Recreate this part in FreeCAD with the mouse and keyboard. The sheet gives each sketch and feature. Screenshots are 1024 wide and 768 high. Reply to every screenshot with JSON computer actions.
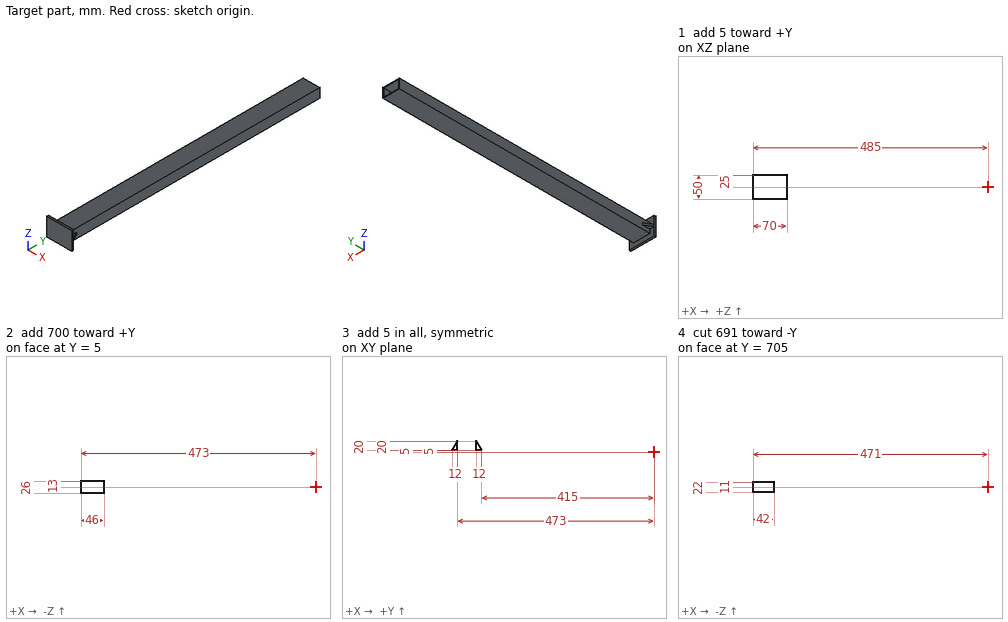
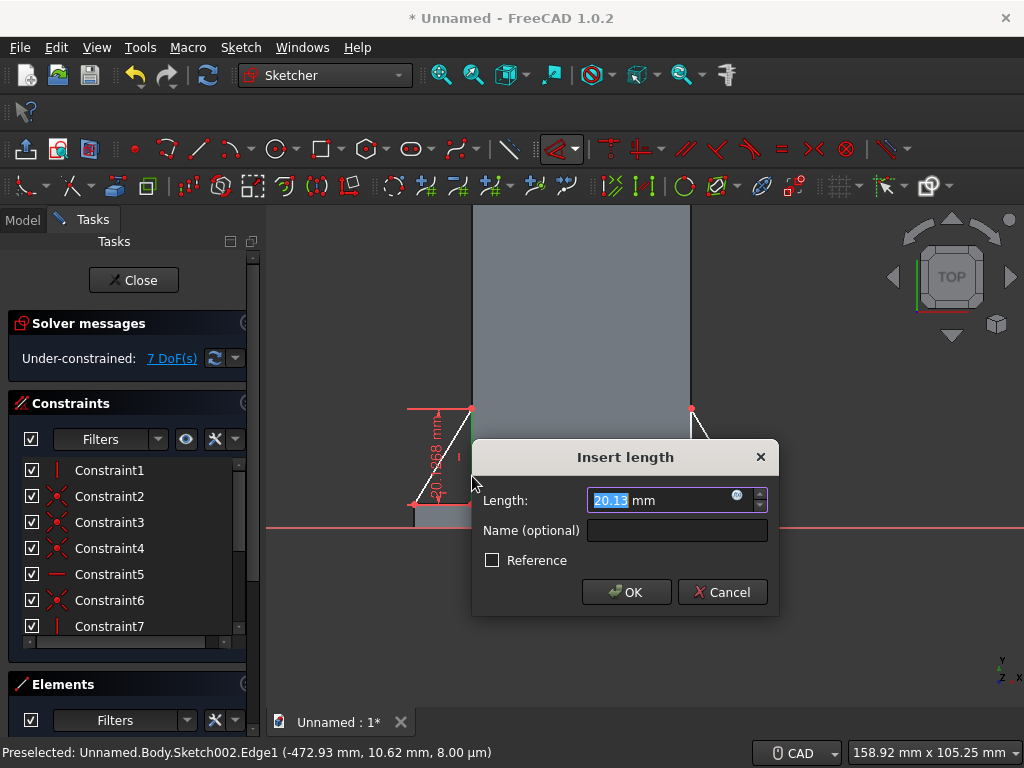
{"action": "type", "text": "20"}
{"action": "key", "text": "Return"}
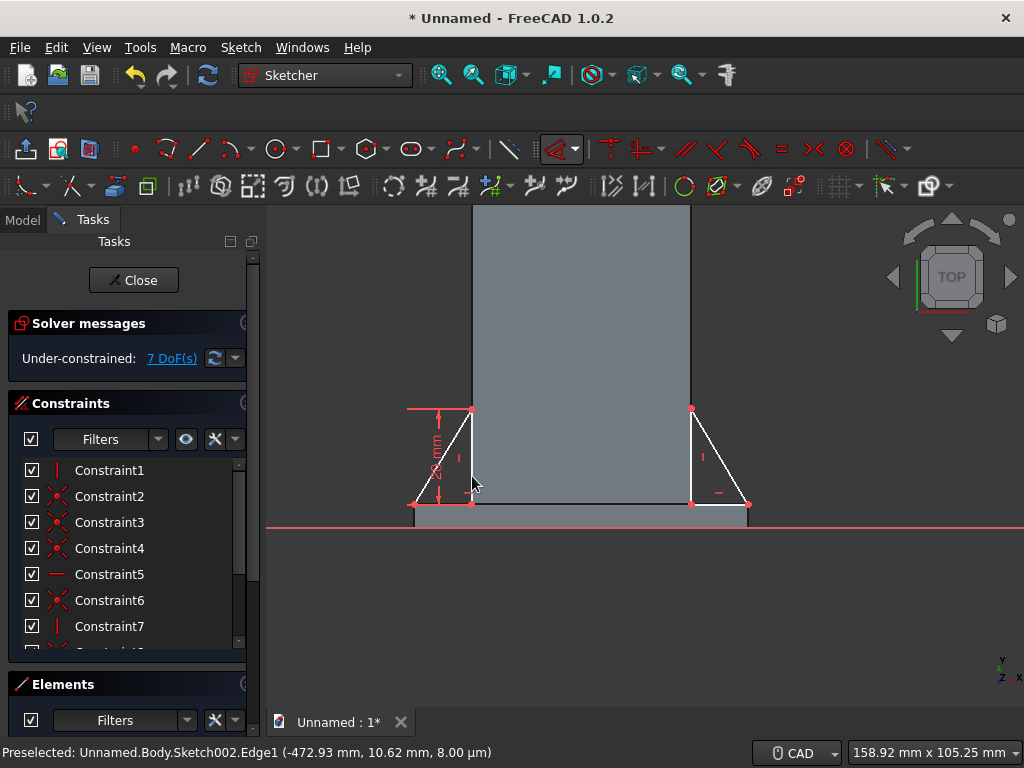
{"action": "left_click", "coordinate": [431, 505]}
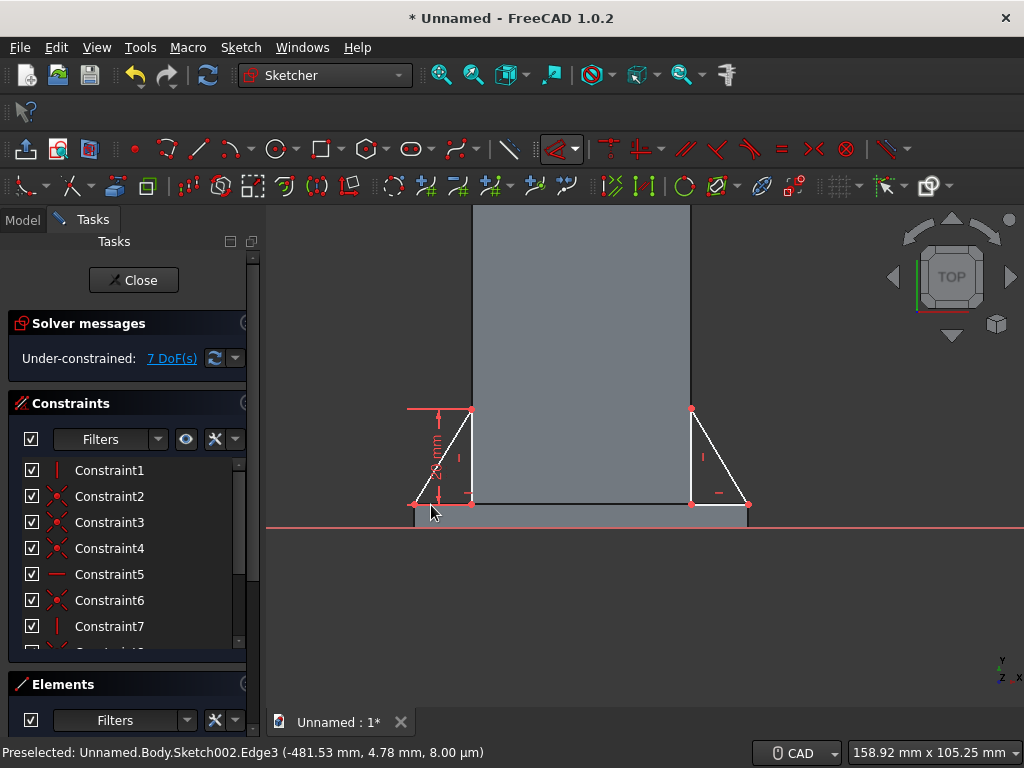
{"action": "key", "text": "l"}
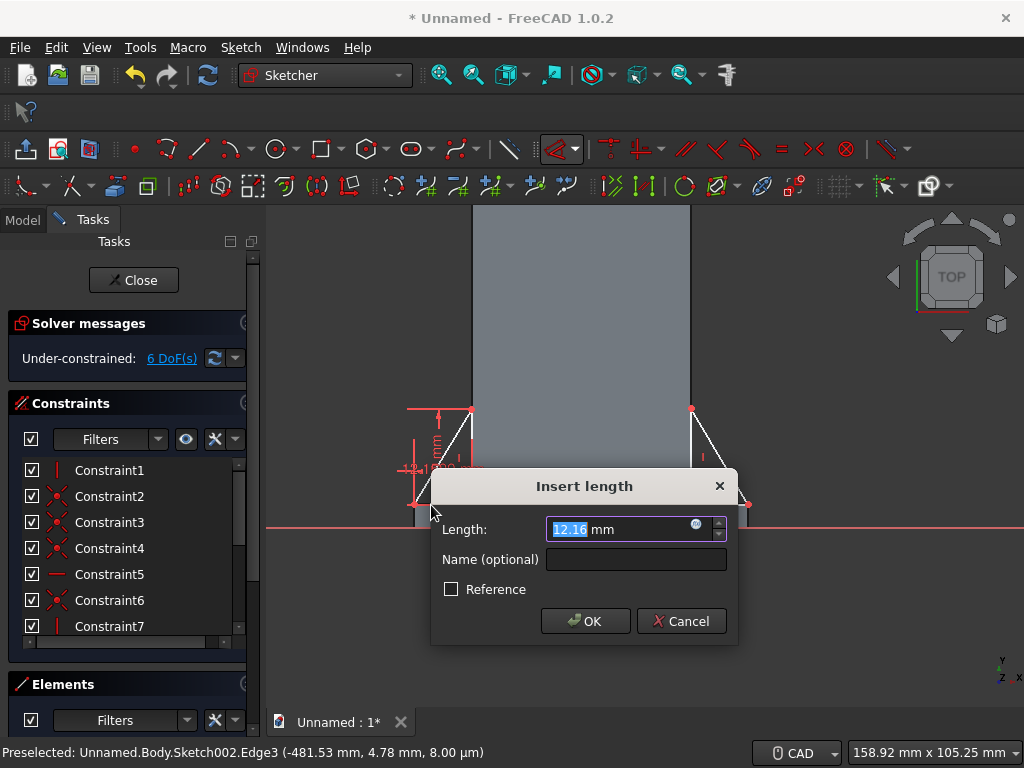
{"action": "type", "text": "12"}
{"action": "key", "text": "Return"}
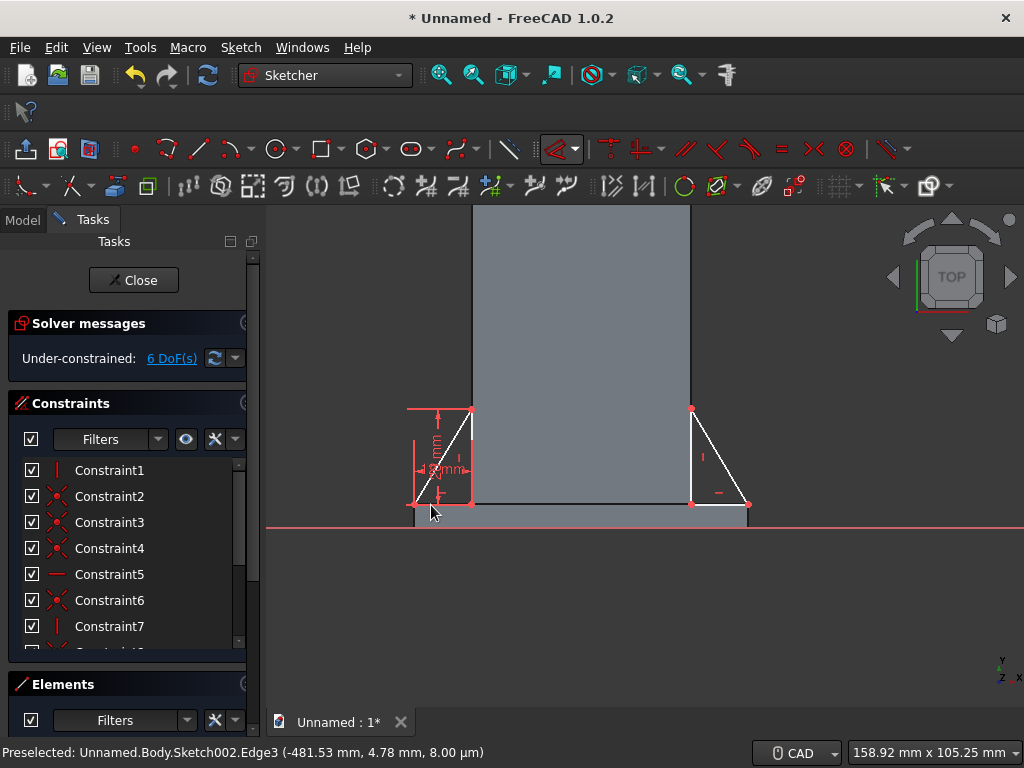
{"action": "left_click", "coordinate": [691, 438]}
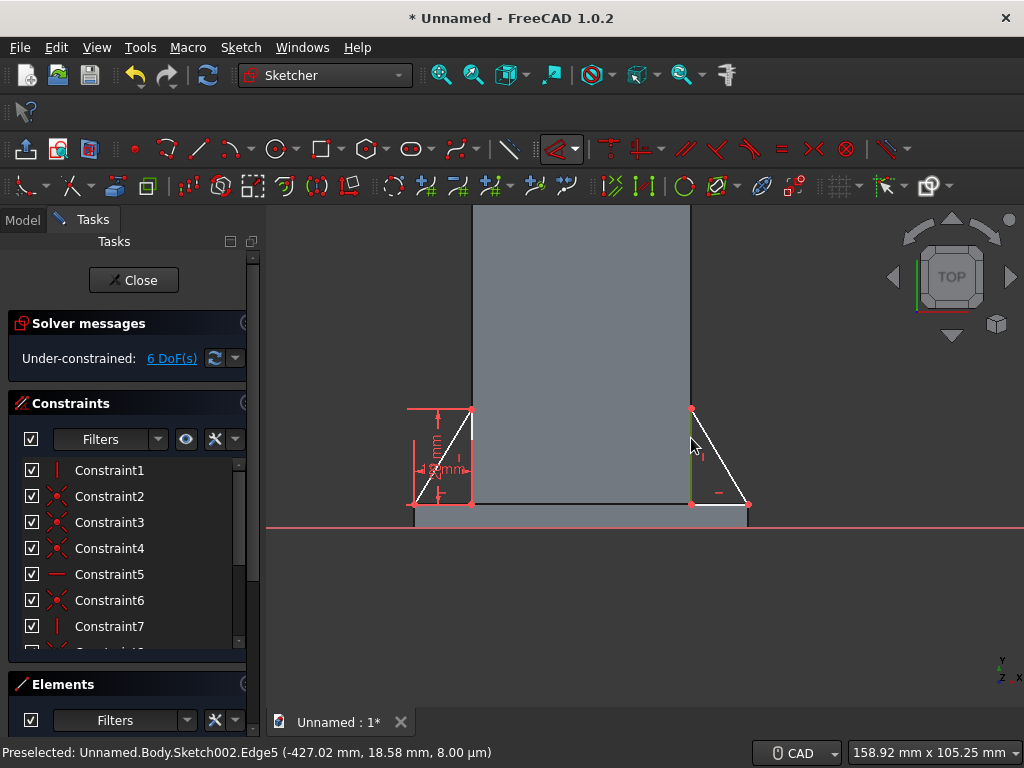
{"action": "left_click", "coordinate": [578, 150]}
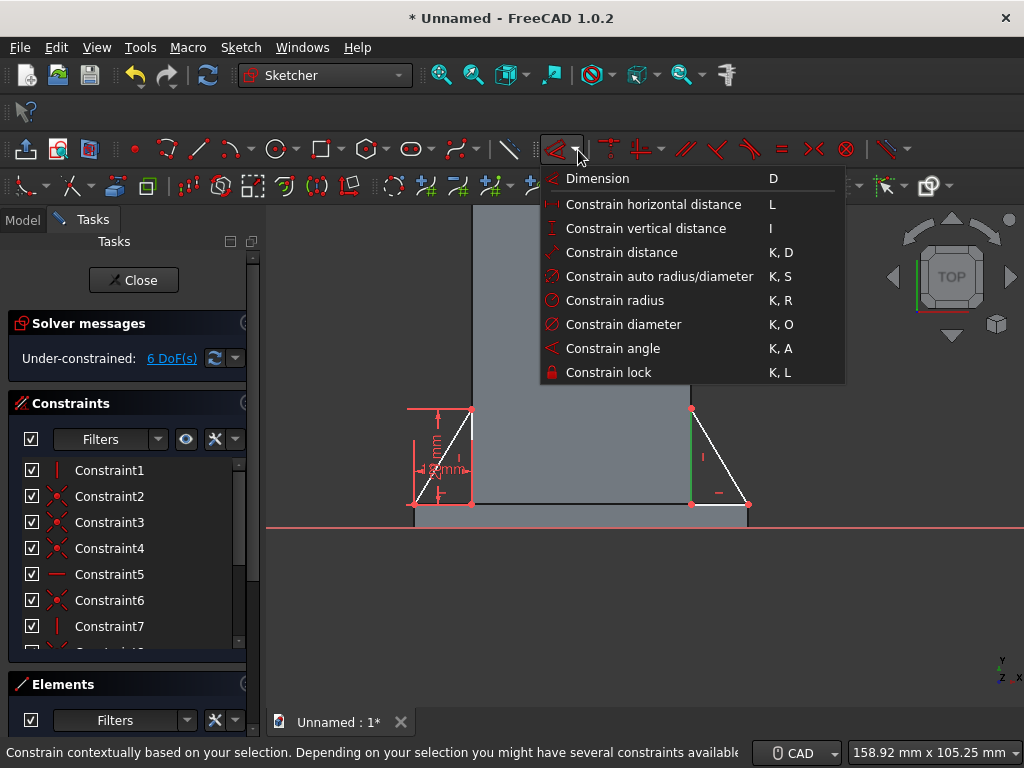
{"action": "left_click", "coordinate": [693, 228]}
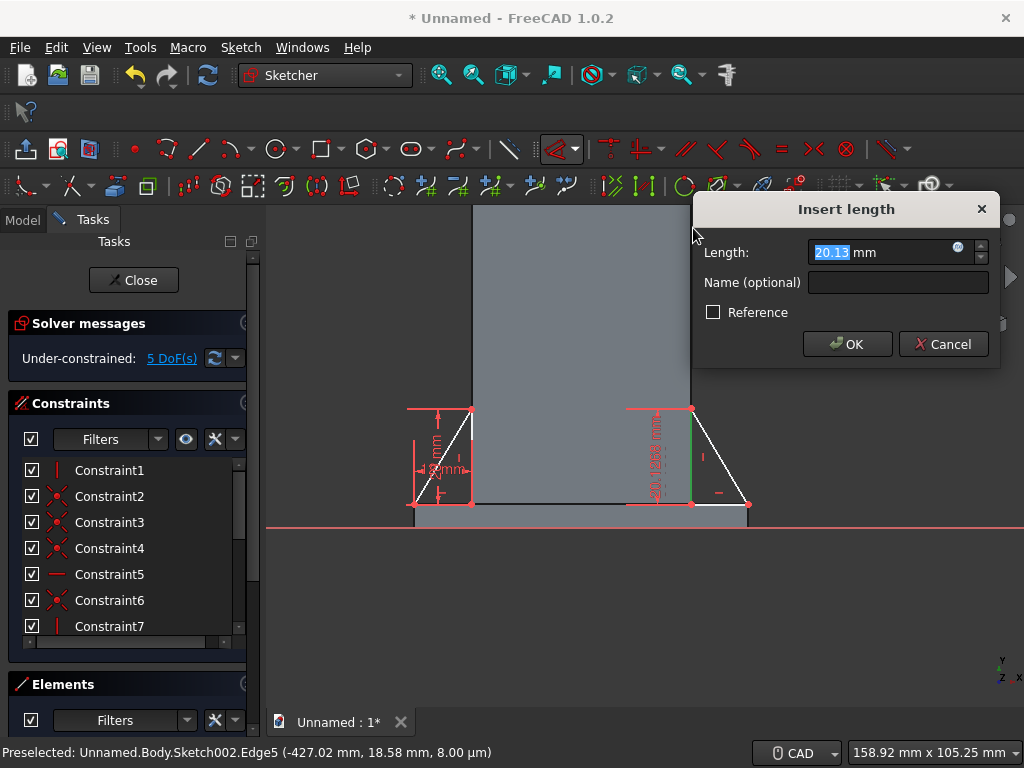
{"action": "type", "text": "20"}
{"action": "key", "text": "Return"}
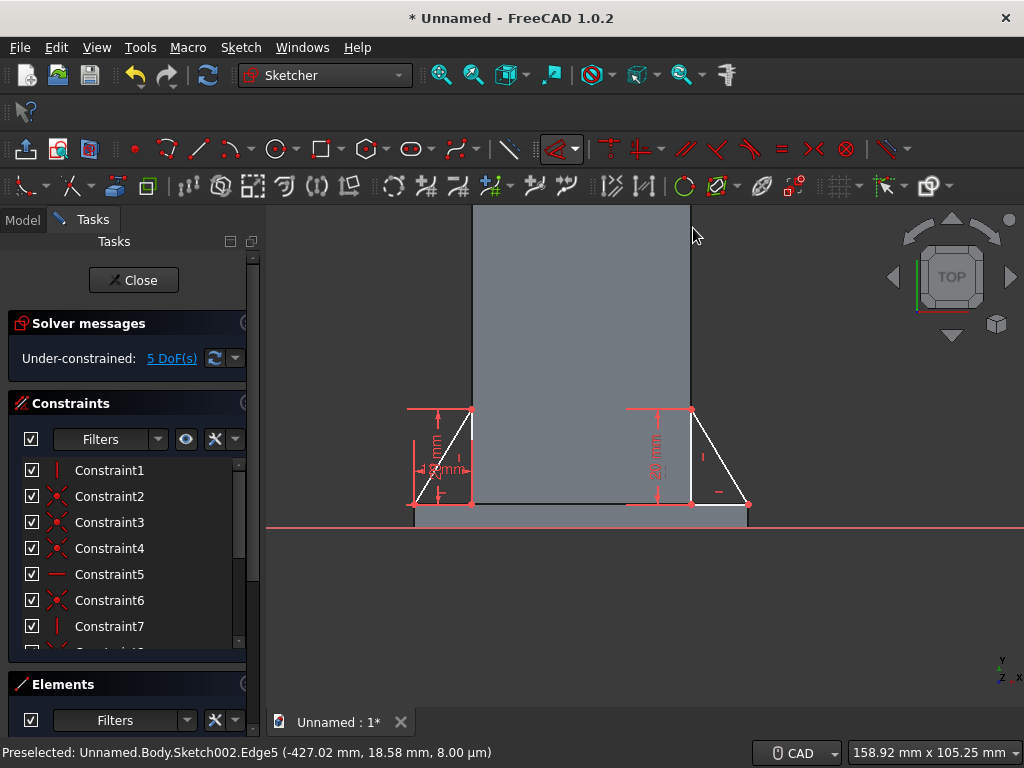
{"action": "left_click", "coordinate": [708, 505]}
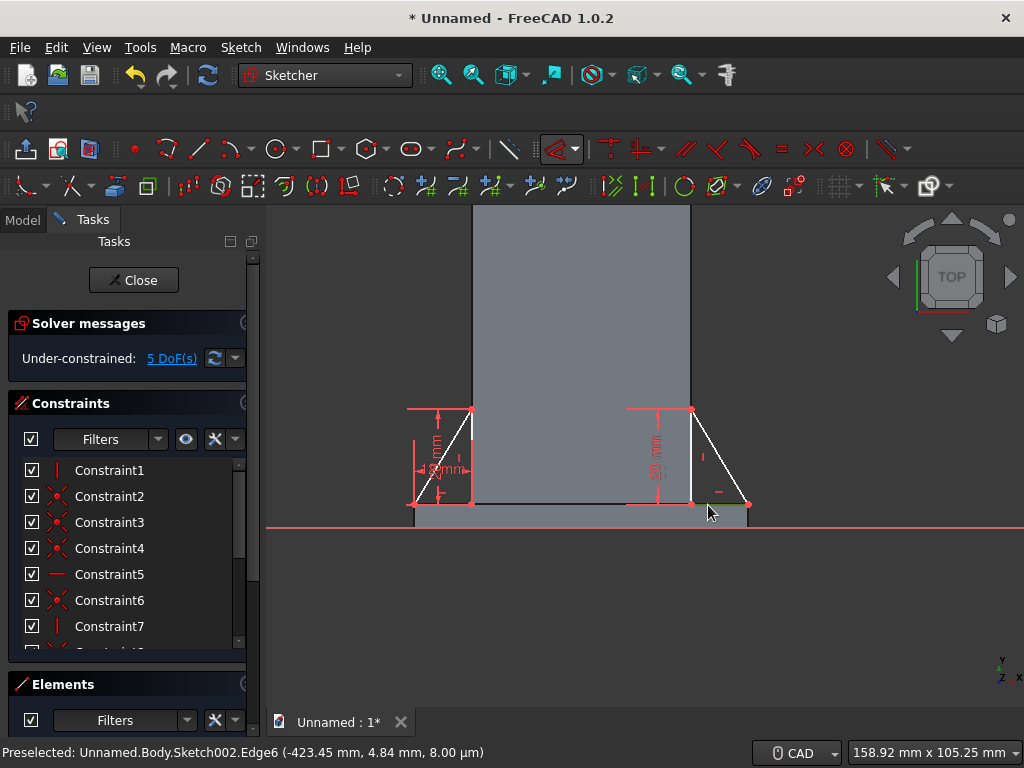
{"action": "left_click", "coordinate": [578, 150]}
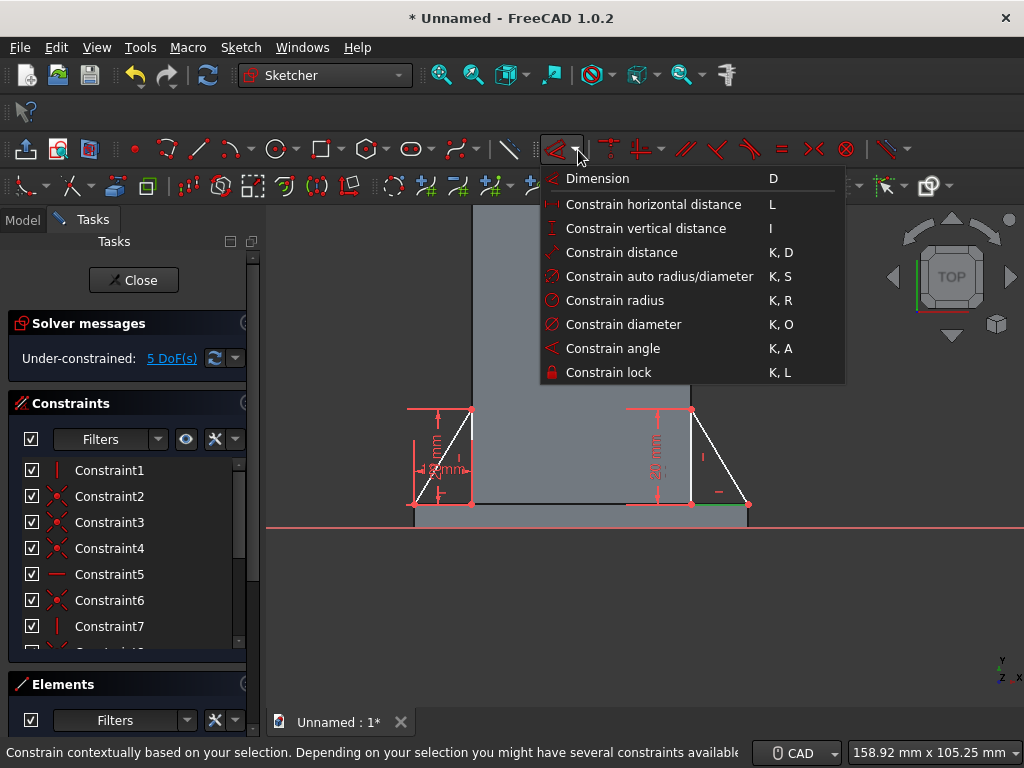
{"action": "left_click", "coordinate": [693, 204]}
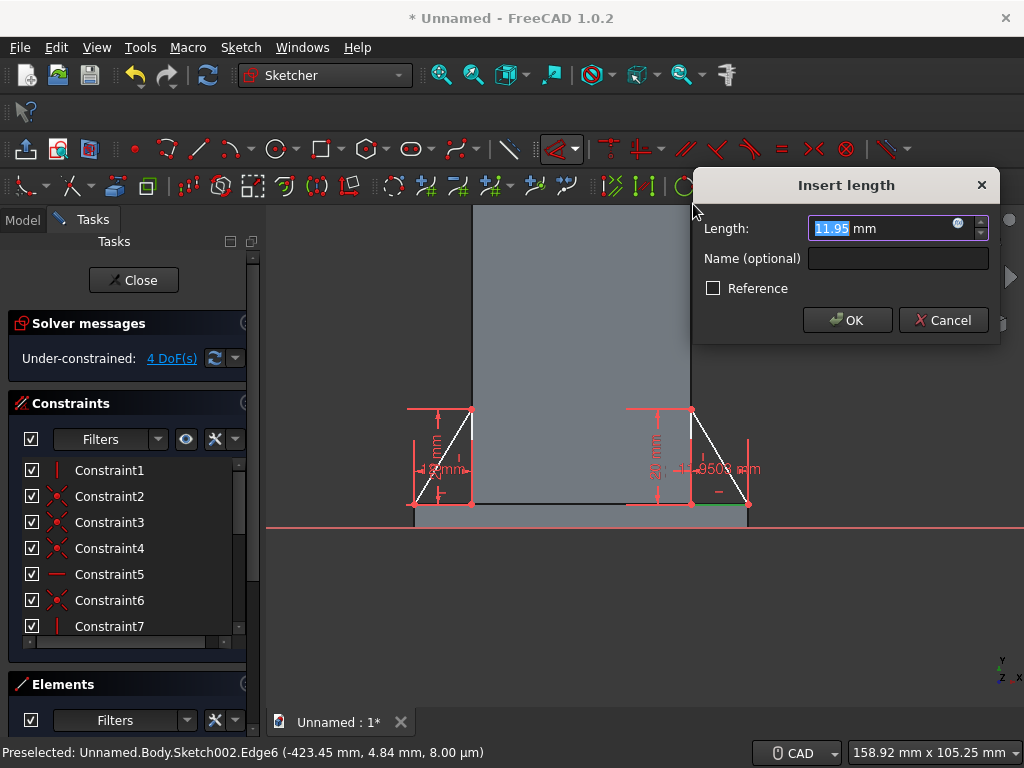
{"action": "type", "text": "12"}
{"action": "key", "text": "Return"}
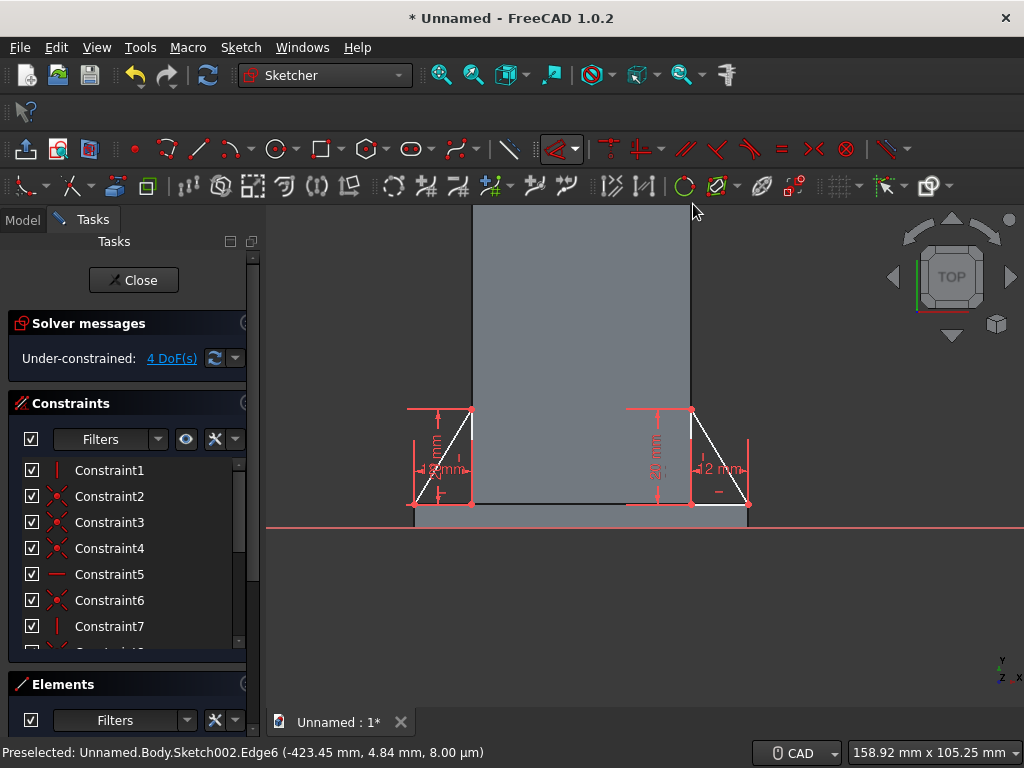
{"action": "scroll", "coordinate": [472, 505], "scroll_direction": "up", "scroll_amount": 3}